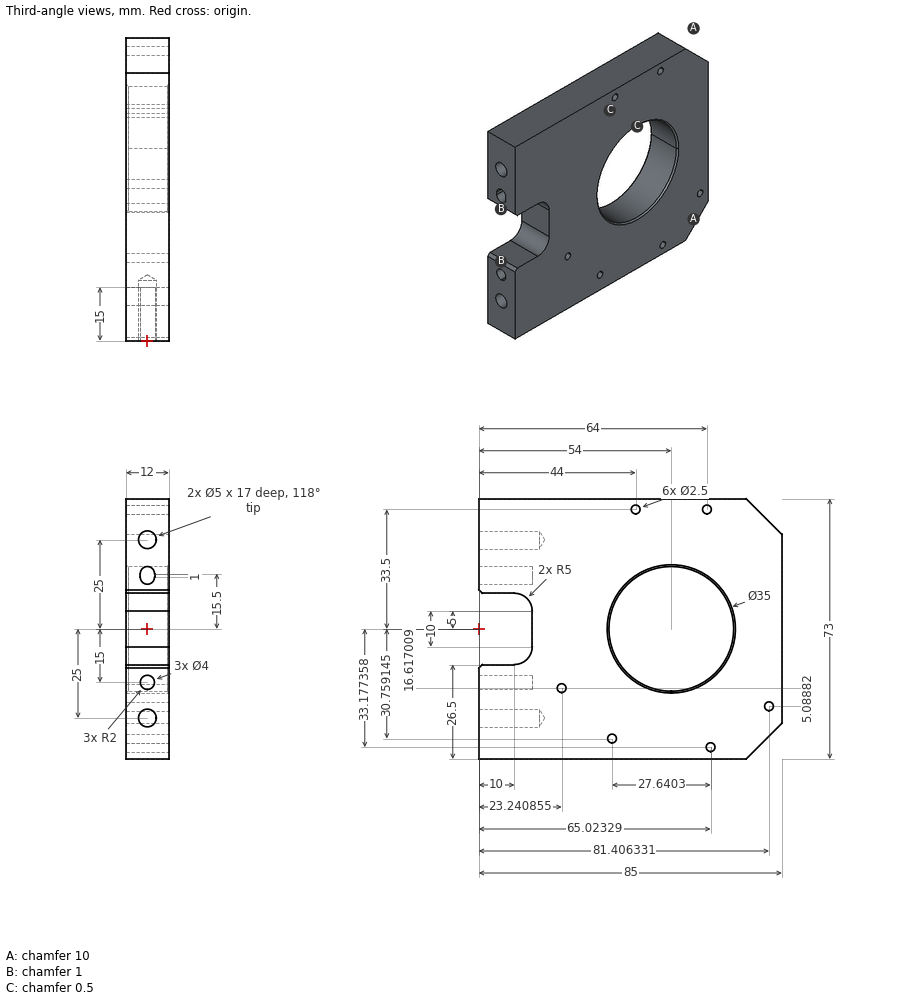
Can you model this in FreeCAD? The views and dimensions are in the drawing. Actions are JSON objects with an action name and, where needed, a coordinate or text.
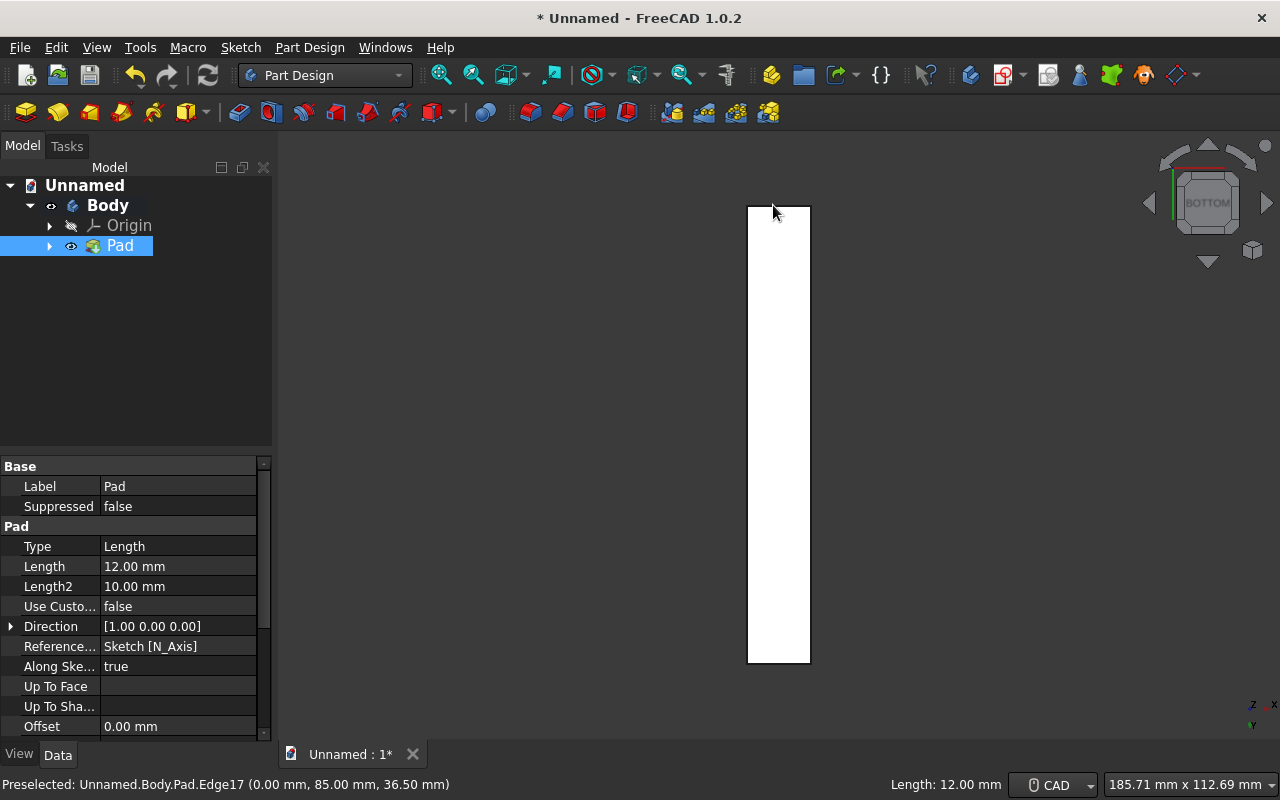
{"action": "left_click", "coordinate": [779, 663], "text": "ctrl"}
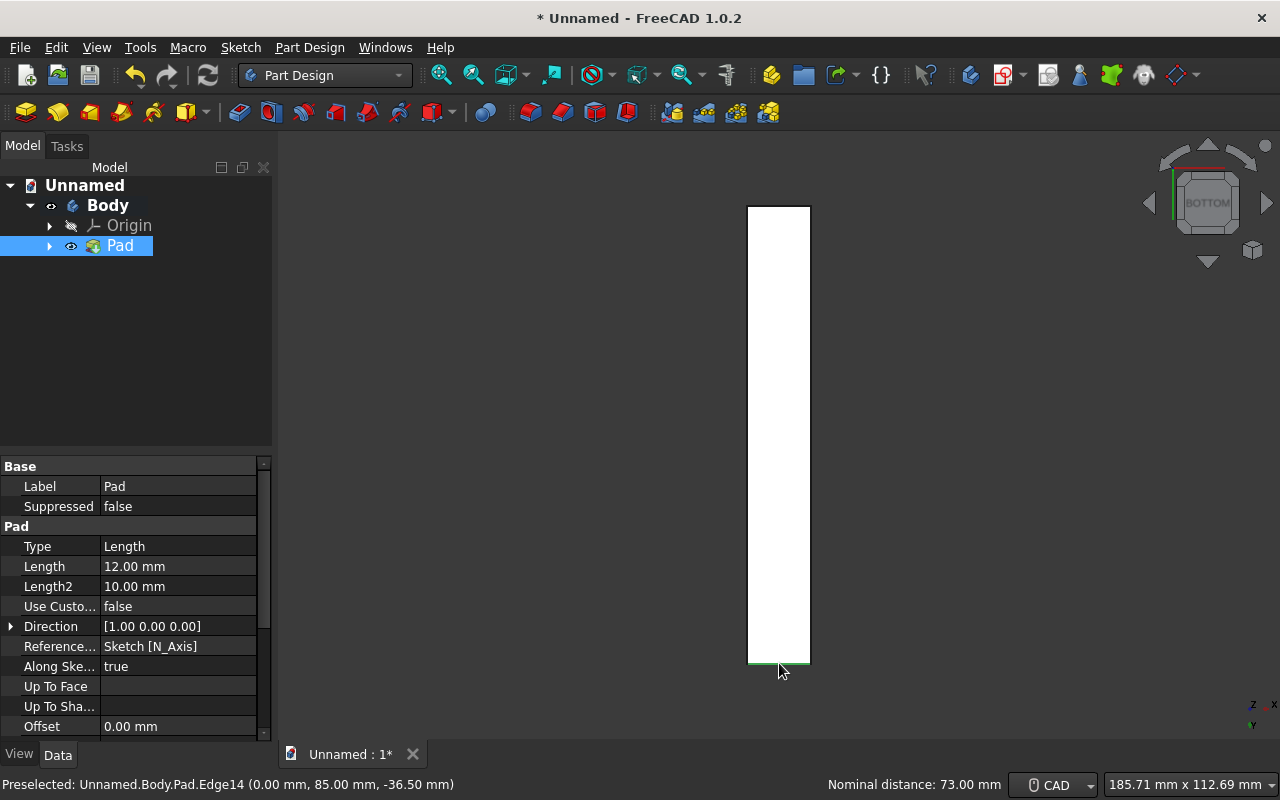
{"action": "left_click", "coordinate": [564, 112]}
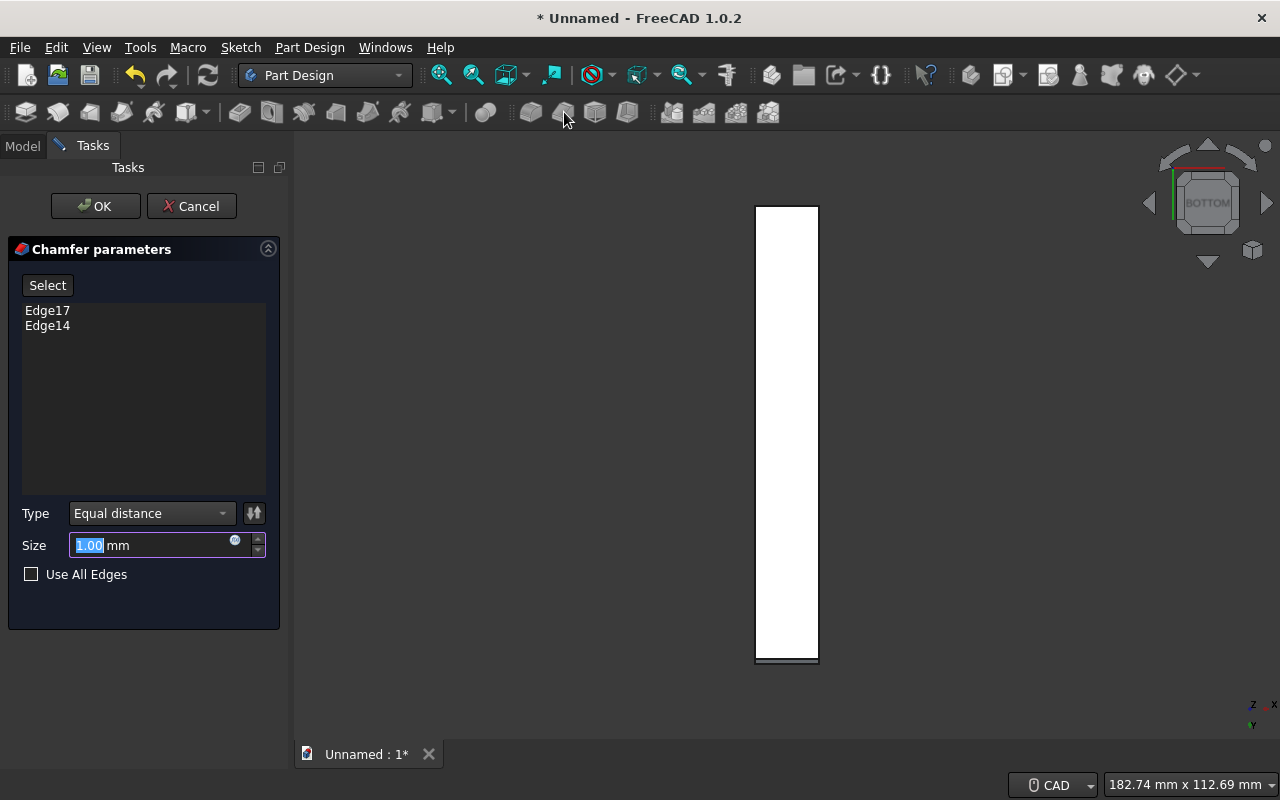
{"action": "type", "text": "10"}
{"action": "key", "text": "Tab"}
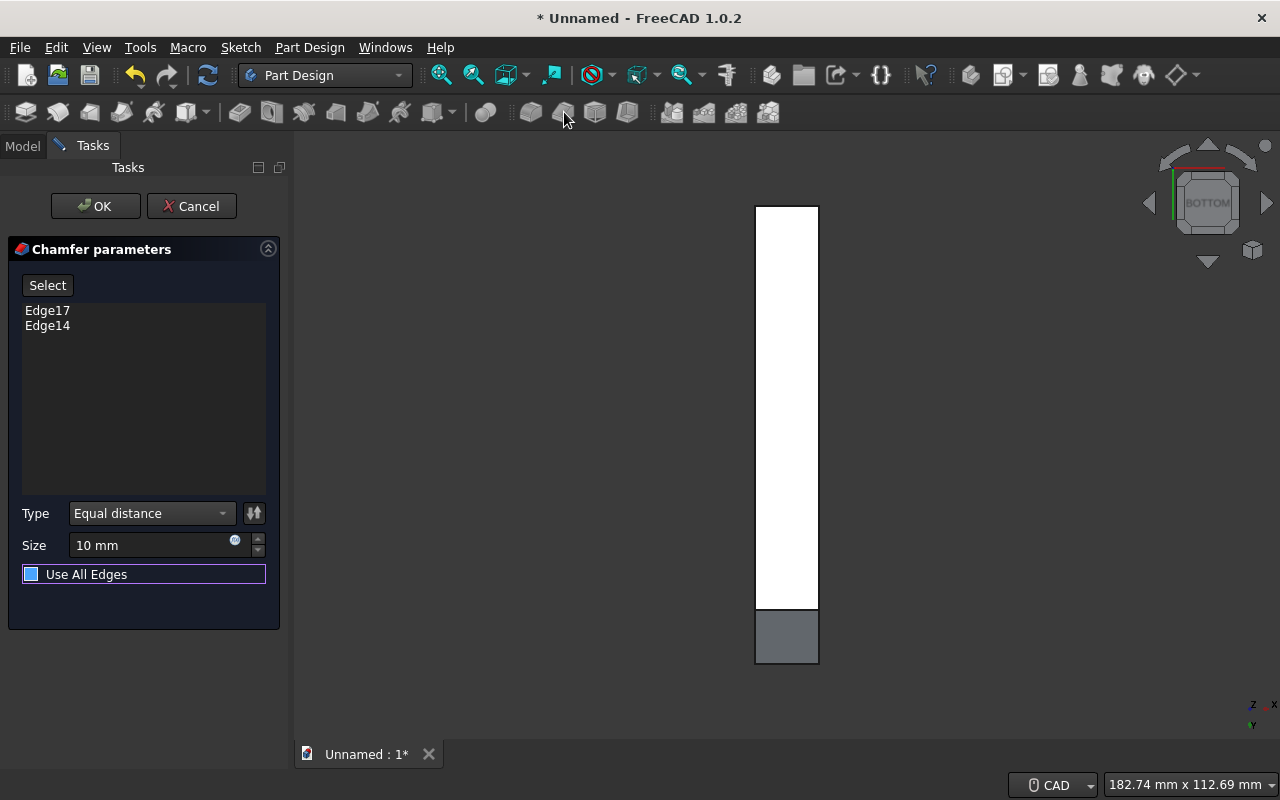
{"action": "left_click", "coordinate": [96, 206]}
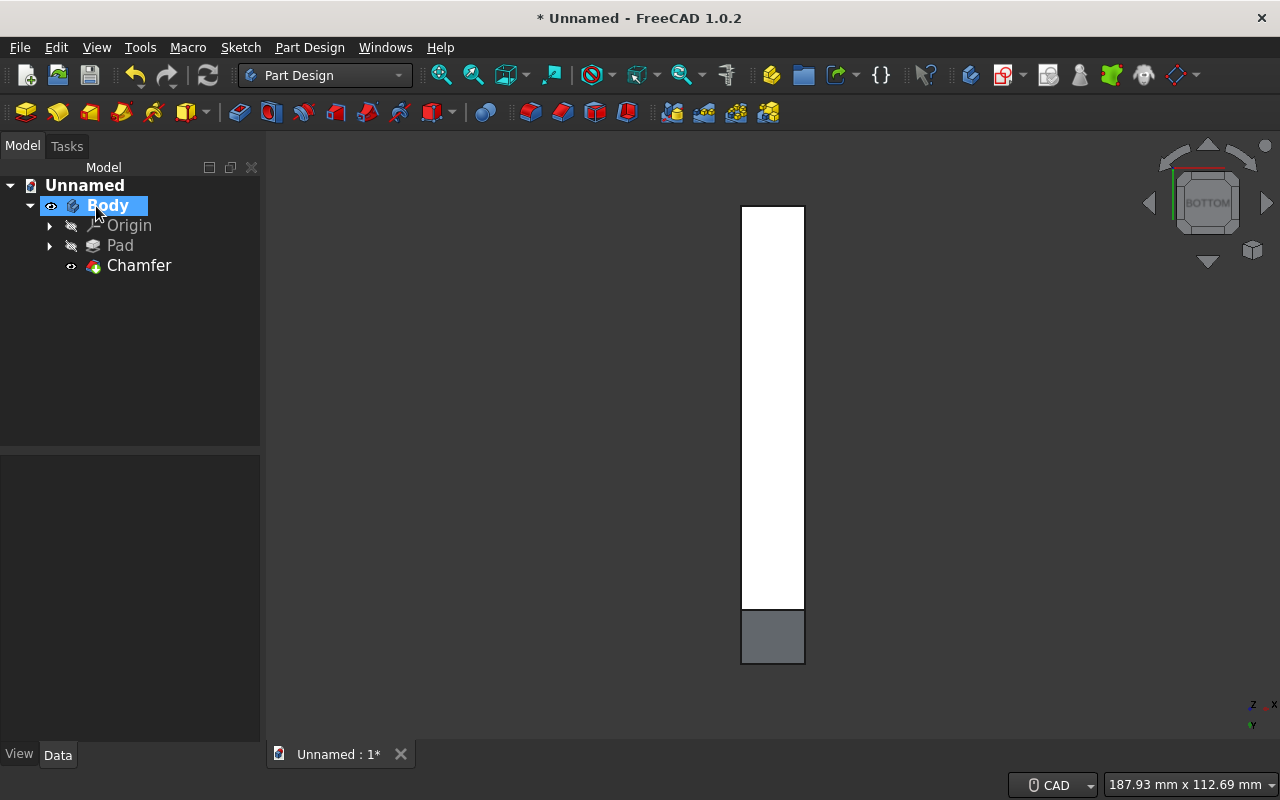
{"action": "key", "text": "0"}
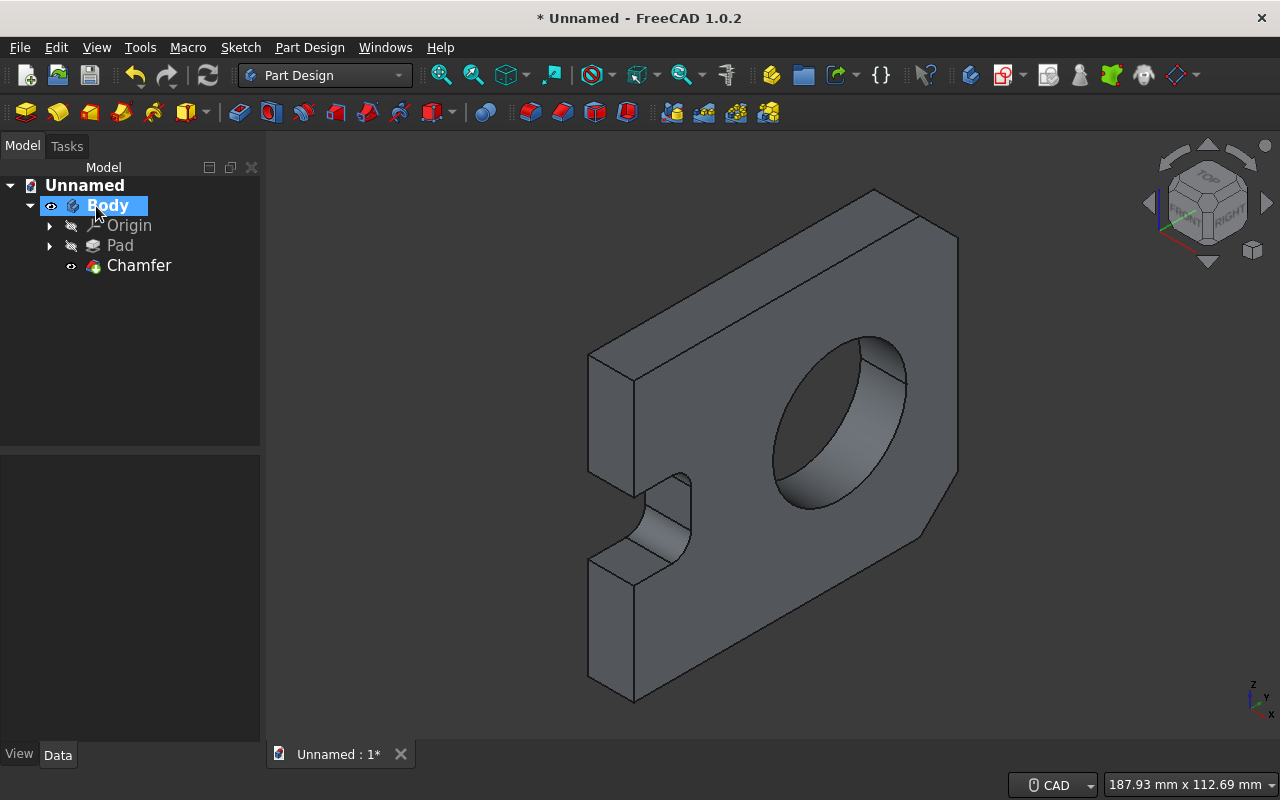
{"action": "left_click", "coordinate": [611, 647]}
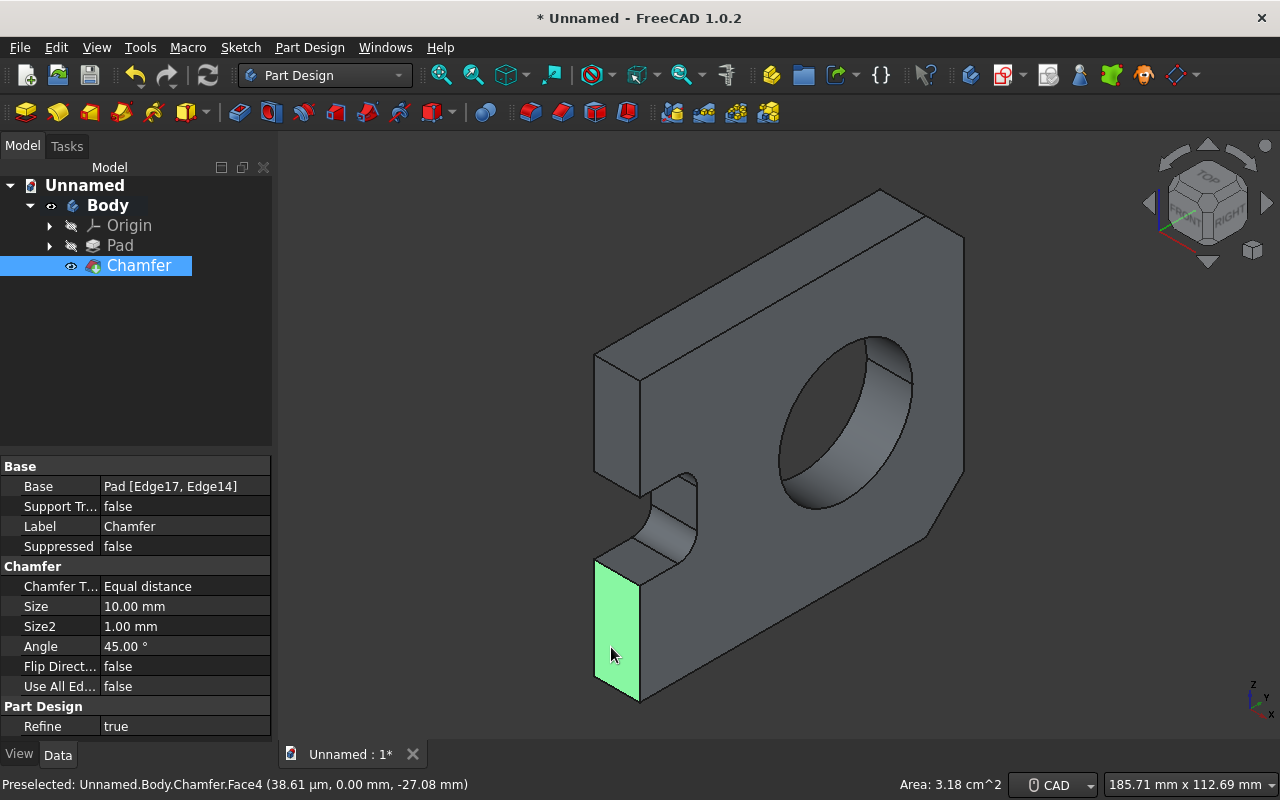
{"action": "left_click", "coordinate": [1004, 76]}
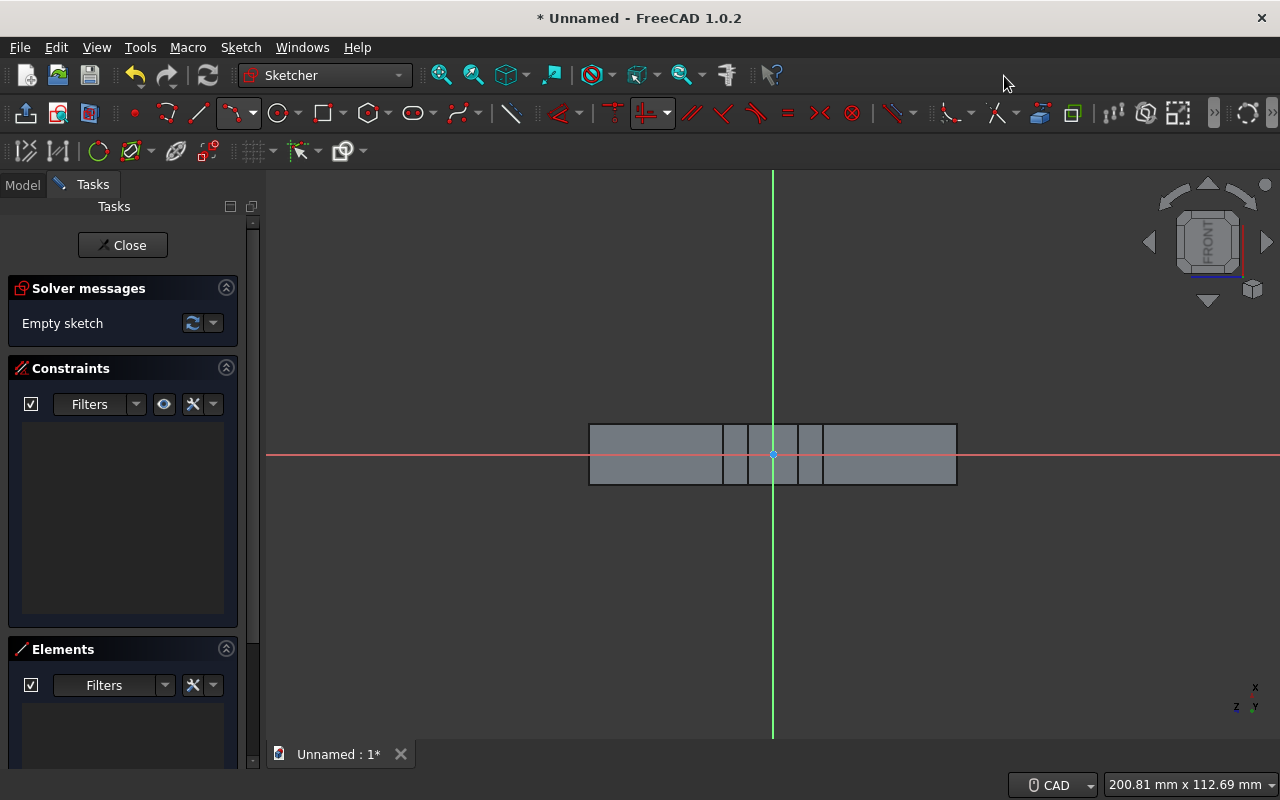
{"action": "scroll", "coordinate": [829, 455], "scroll_direction": "up", "scroll_amount": 4}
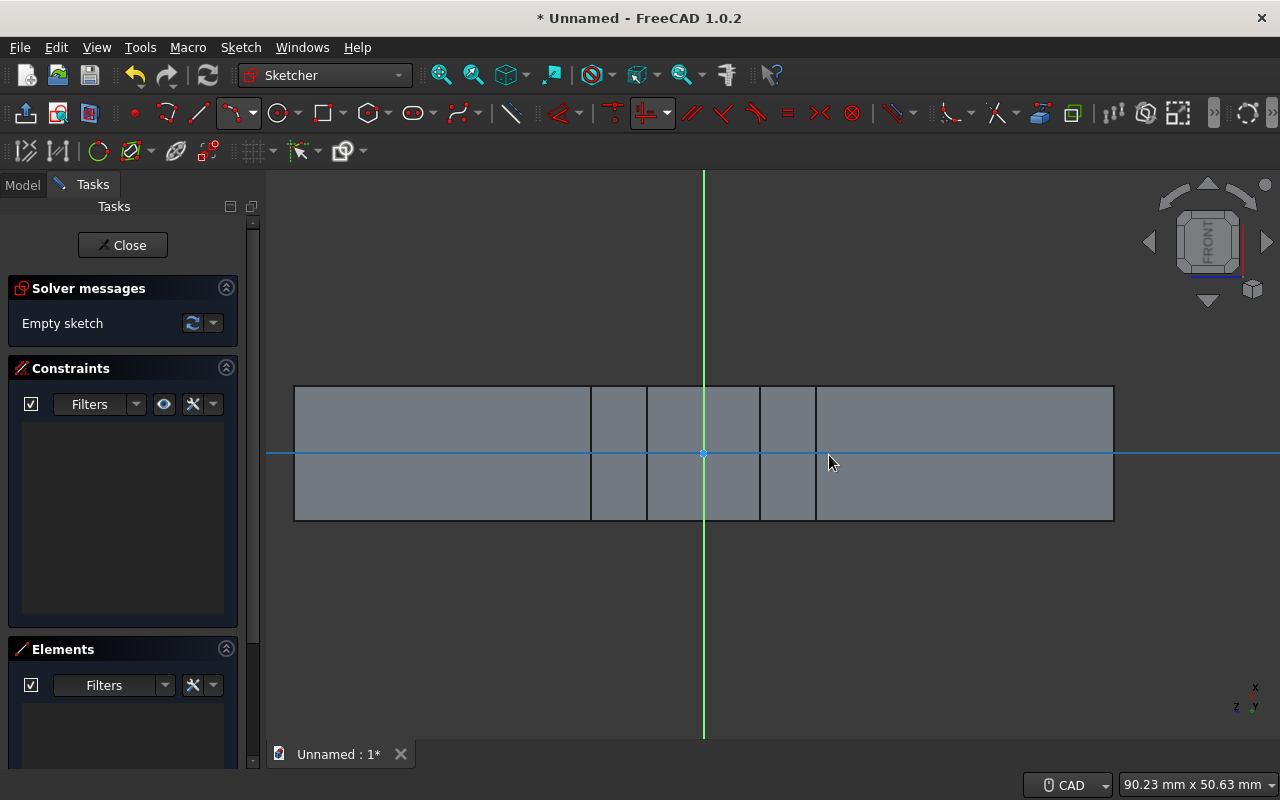
{"action": "left_click", "coordinate": [278, 114]}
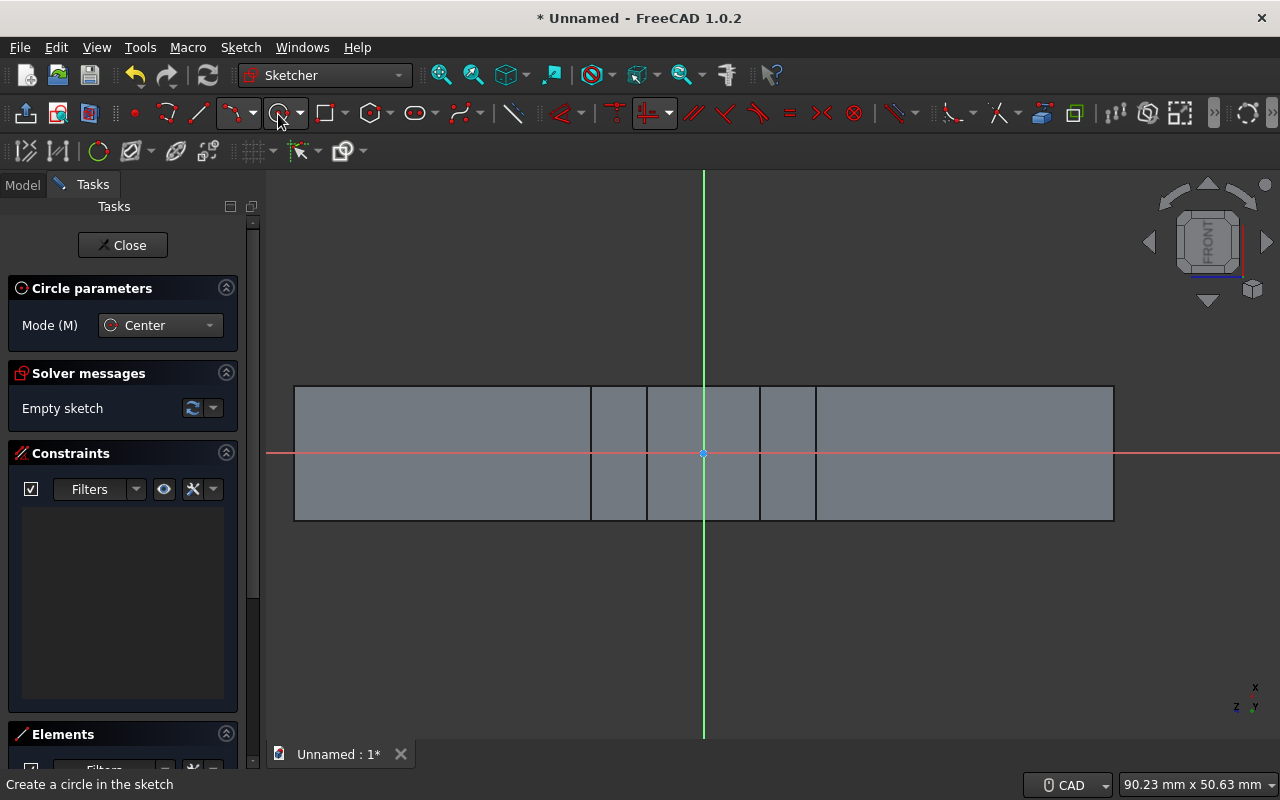
{"action": "left_click", "coordinate": [423, 453]}
{"action": "mouse_move", "coordinate": [443, 433]}